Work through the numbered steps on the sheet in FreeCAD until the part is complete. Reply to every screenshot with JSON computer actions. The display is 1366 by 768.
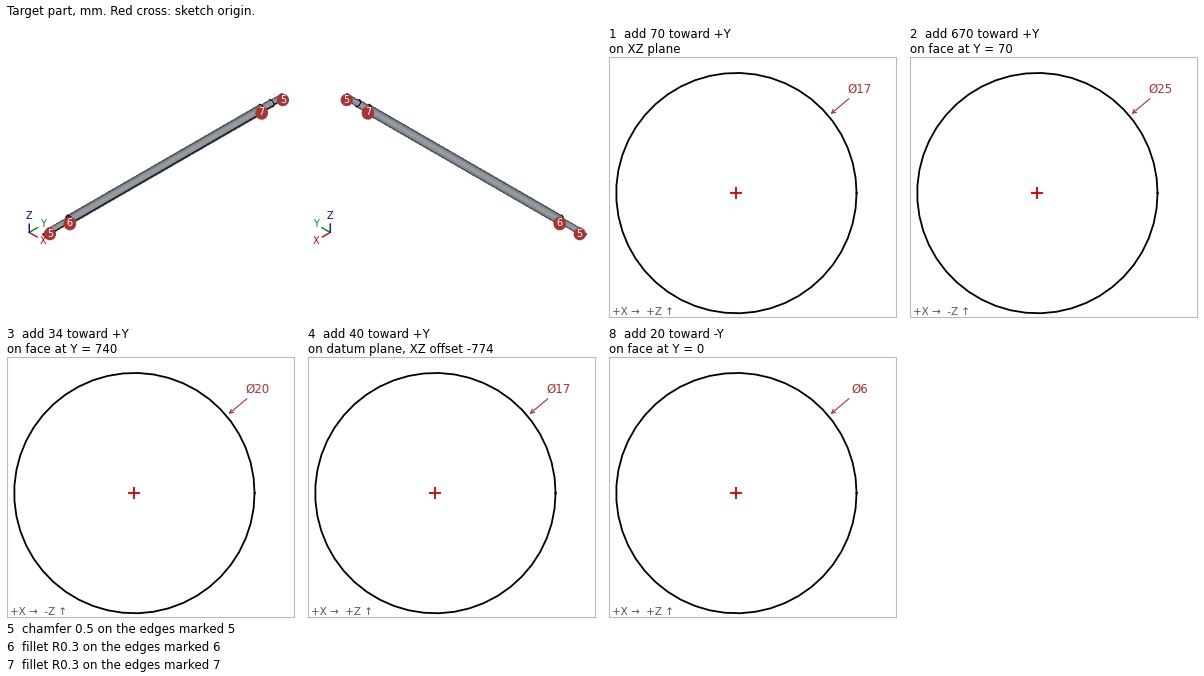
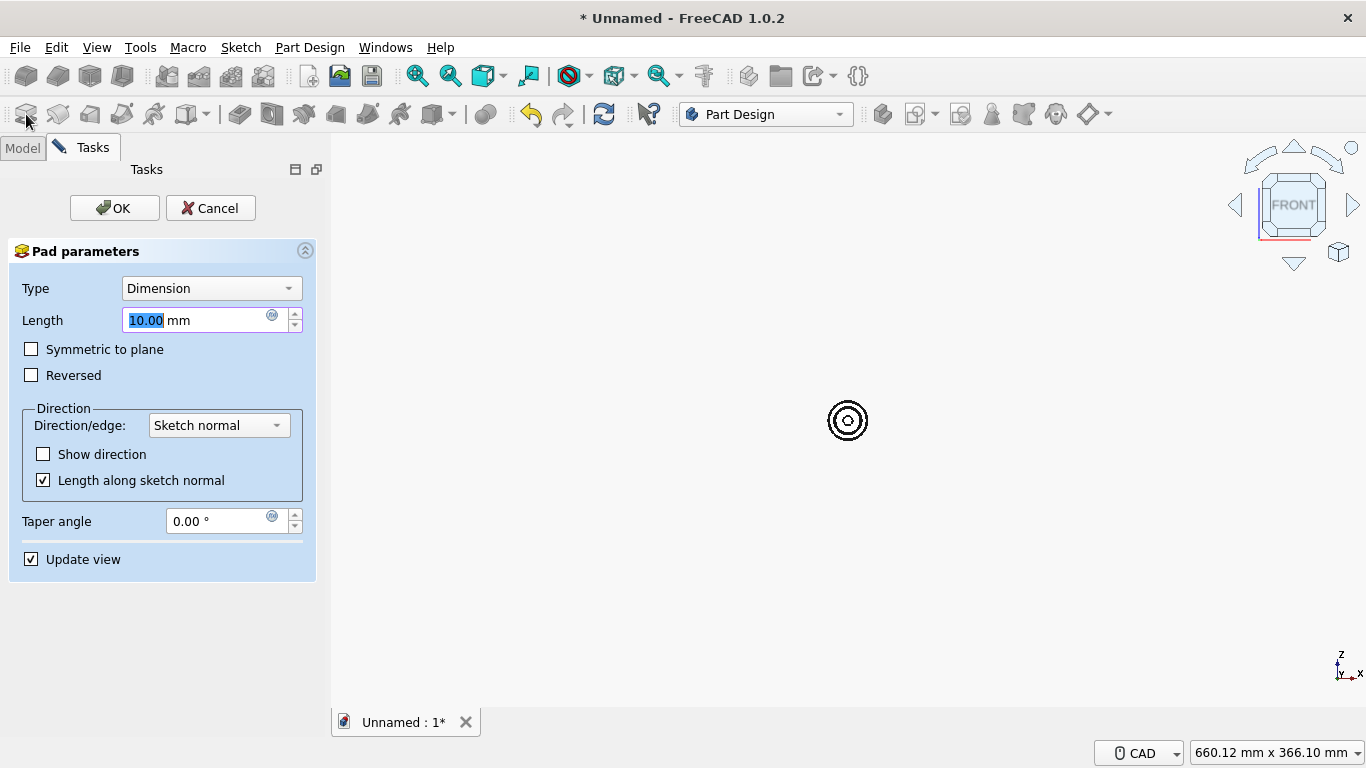
{"action": "type", "text": "20"}
{"action": "key", "text": "Tab"}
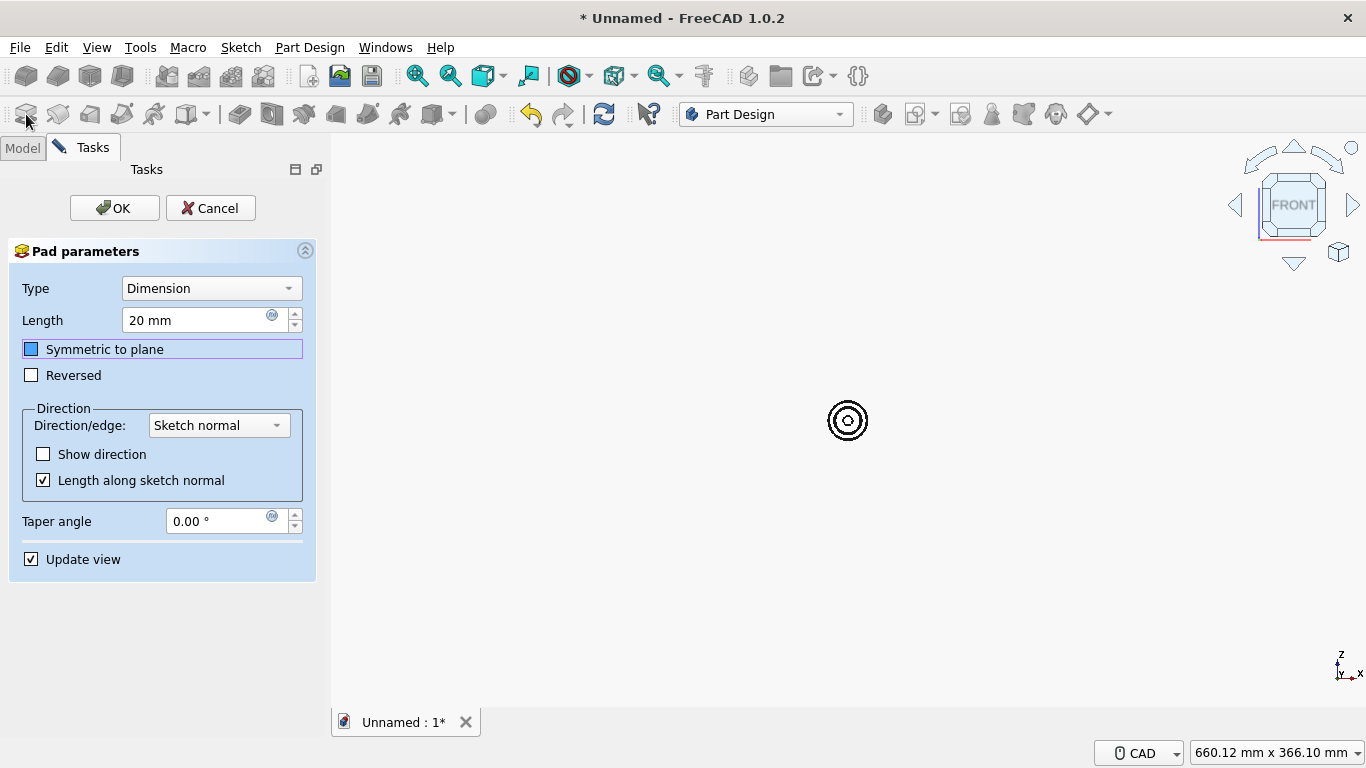
{"action": "left_click", "coordinate": [115, 208]}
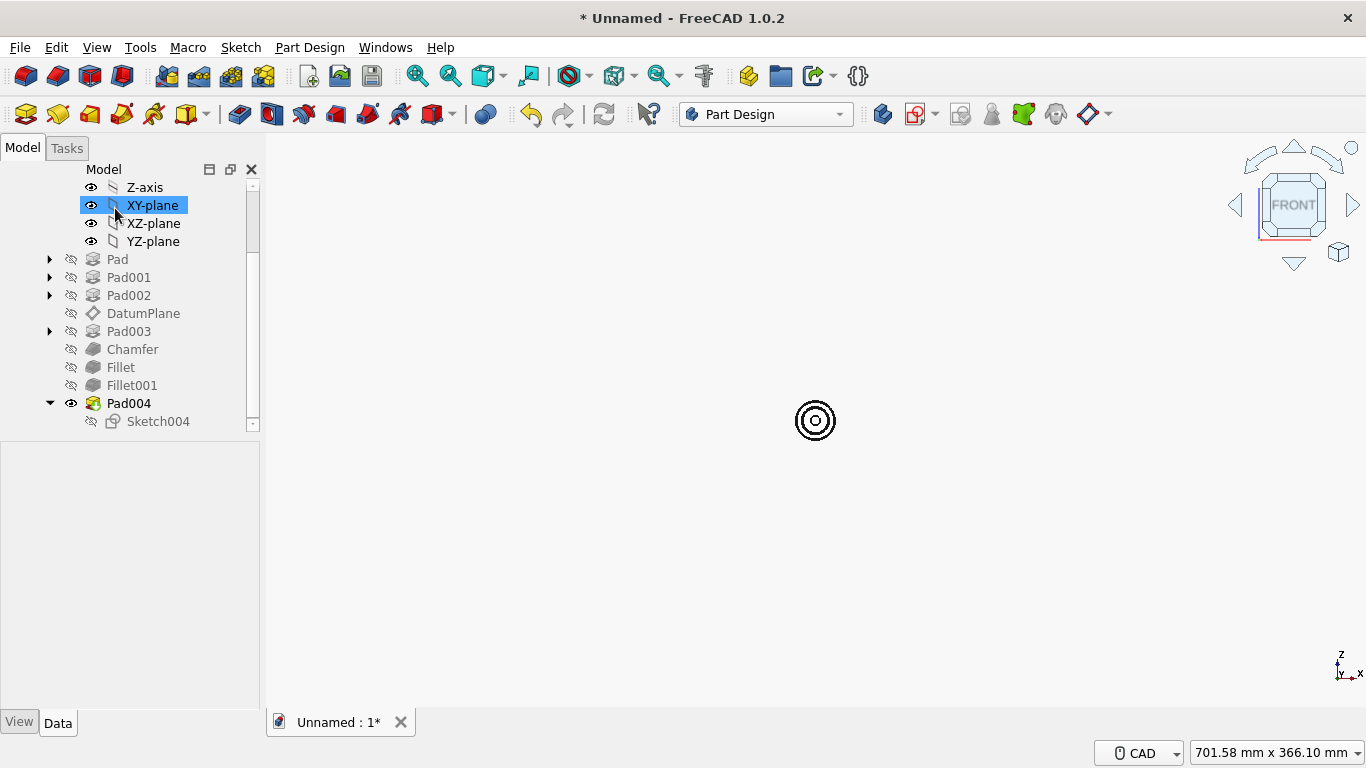
{"action": "key", "text": "0"}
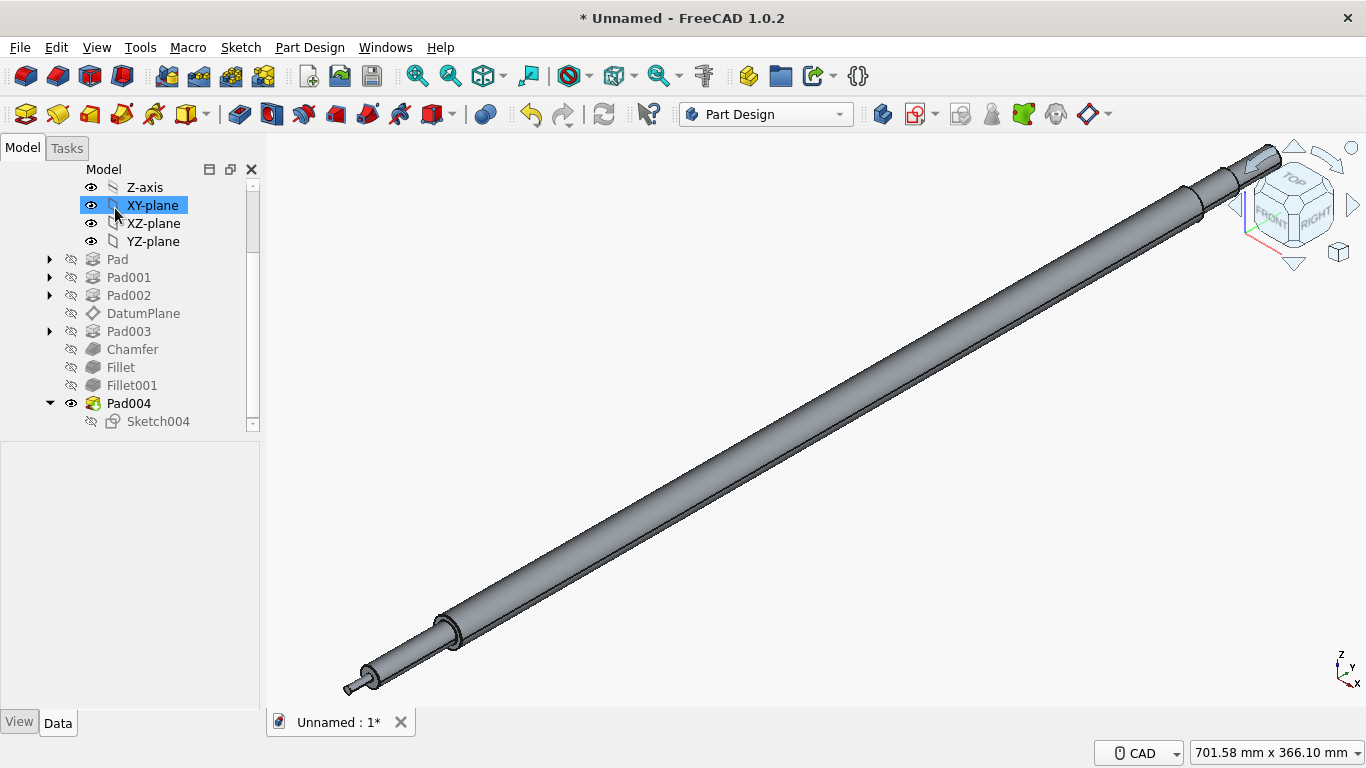
{"action": "left_click", "coordinate": [418, 76]}